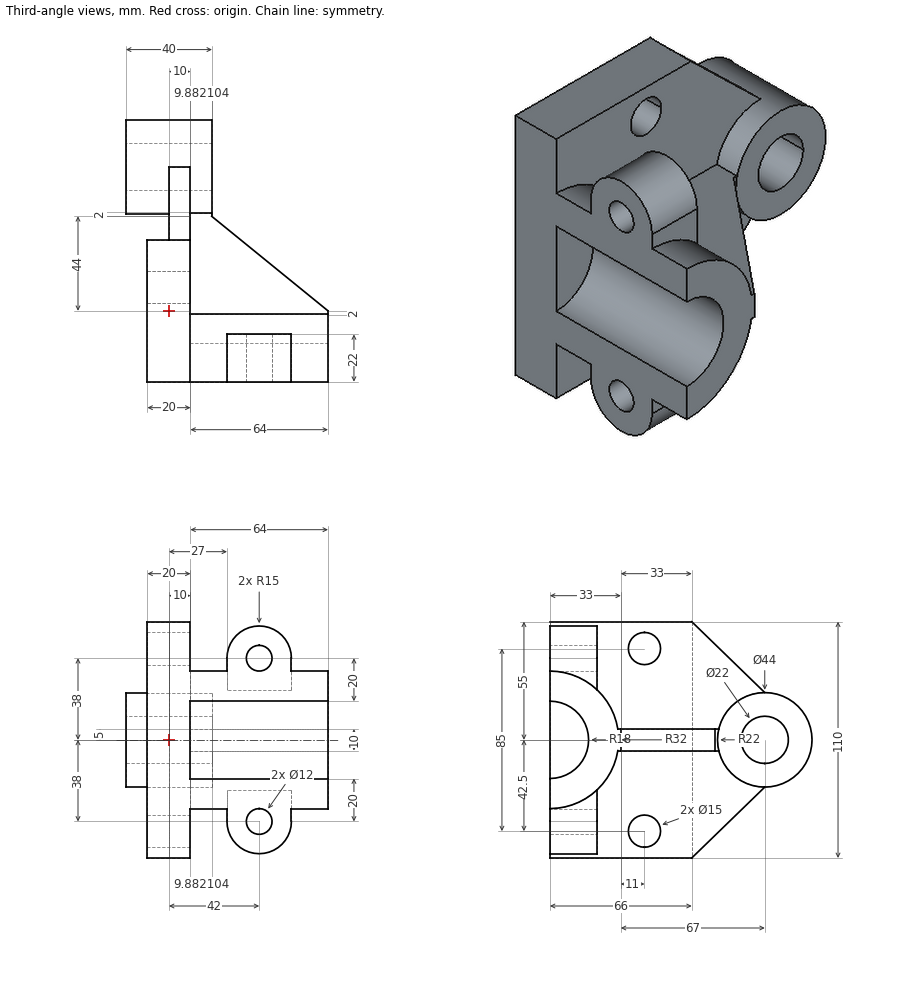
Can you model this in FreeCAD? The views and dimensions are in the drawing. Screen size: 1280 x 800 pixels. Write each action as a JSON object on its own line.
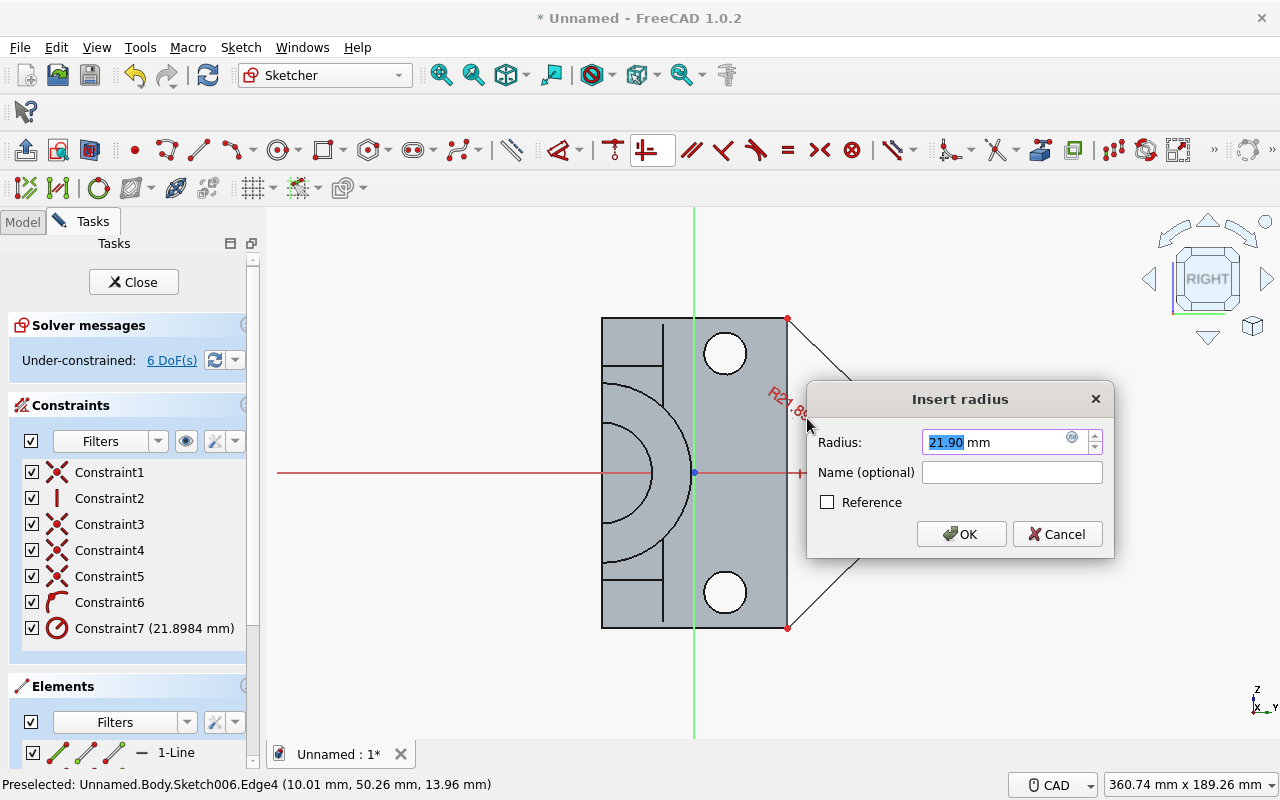
{"action": "type", "text": "22"}
{"action": "key", "text": "Return"}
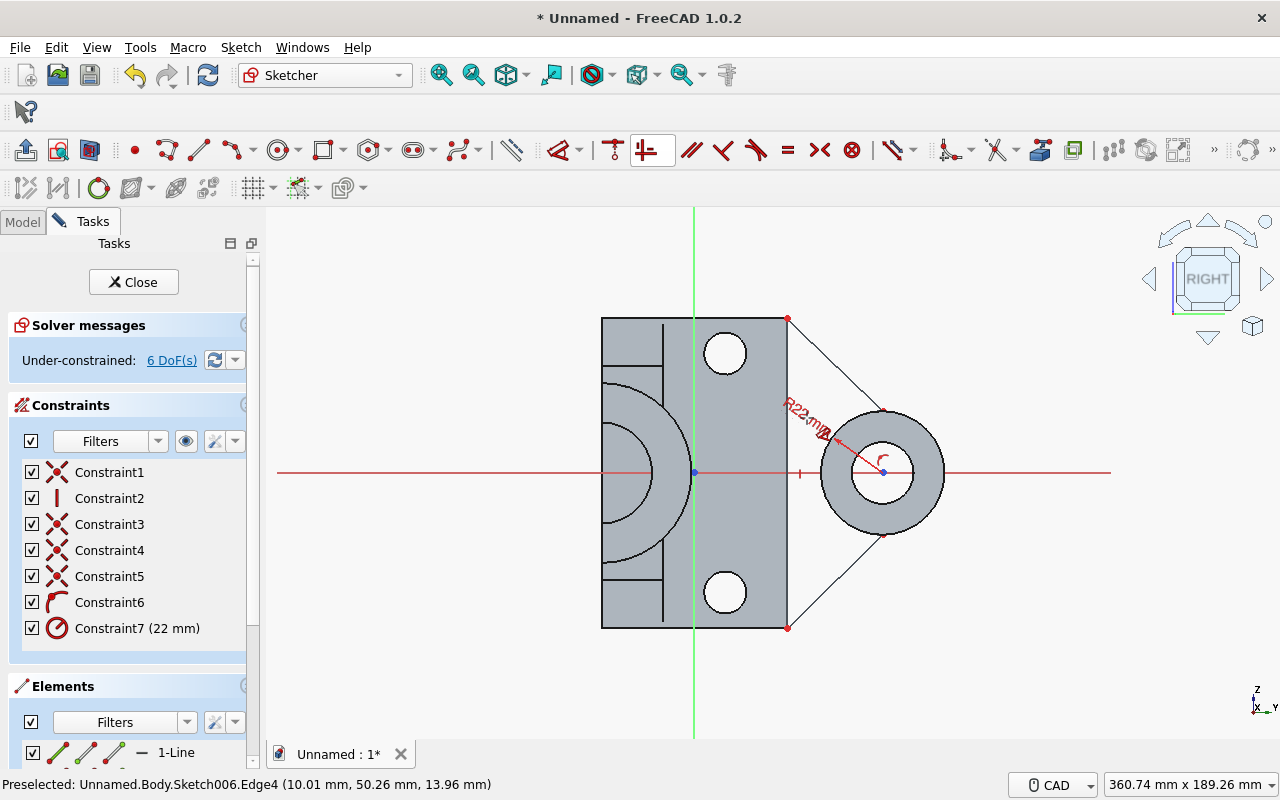
{"action": "left_click", "coordinate": [787, 412]}
{"action": "left_click", "coordinate": [753, 545]}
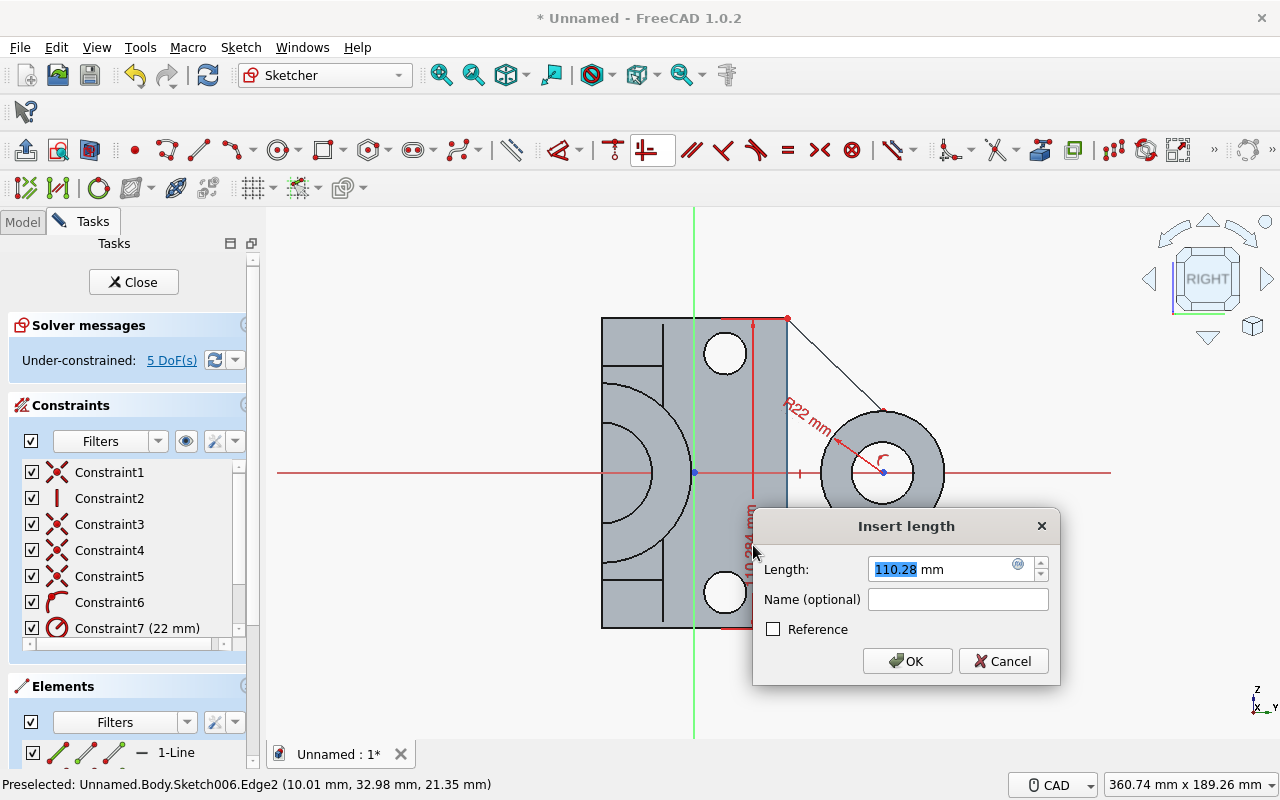
{"action": "type", "text": "110"}
{"action": "key", "text": "Return"}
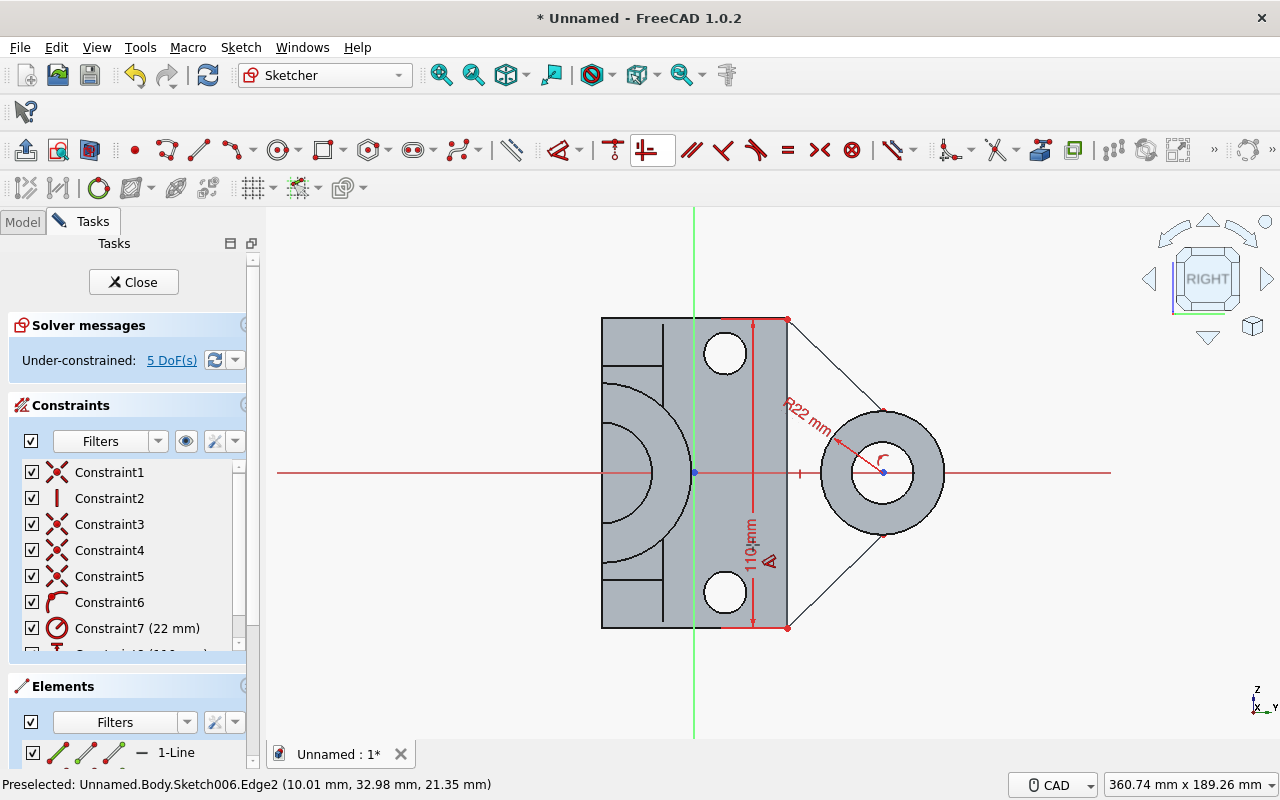
{"action": "left_click", "coordinate": [883, 411]}
{"action": "left_click", "coordinate": [745, 377]}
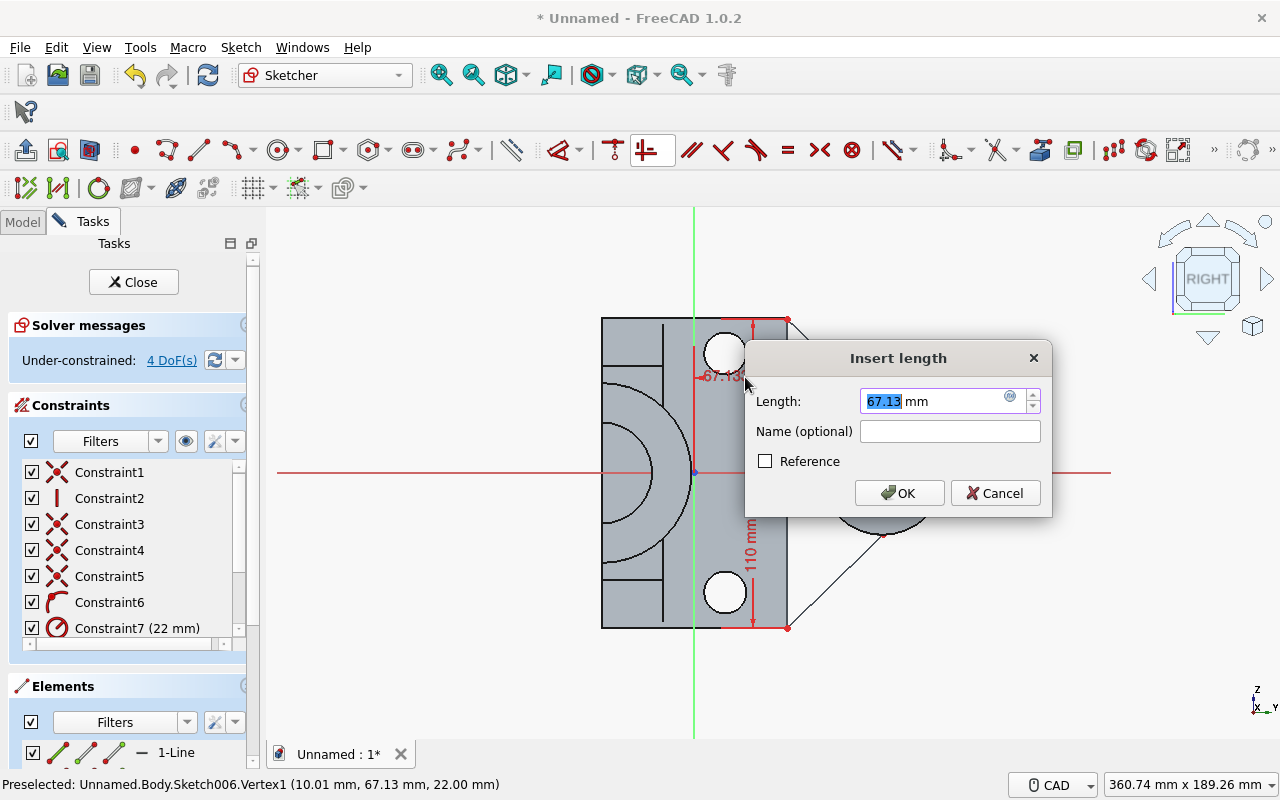
{"action": "type", "text": "67"}
{"action": "key", "text": "Return"}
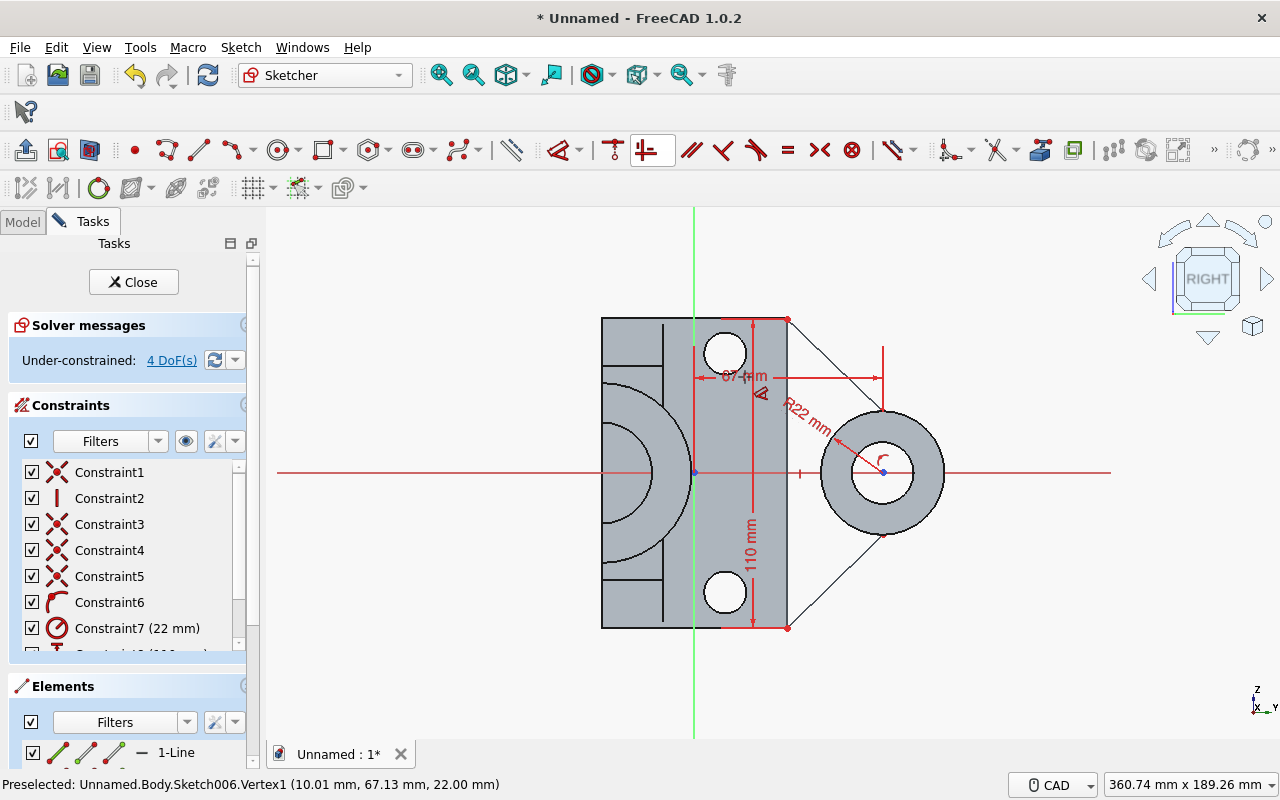
{"action": "left_click", "coordinate": [787, 319]}
{"action": "left_click", "coordinate": [741, 285]}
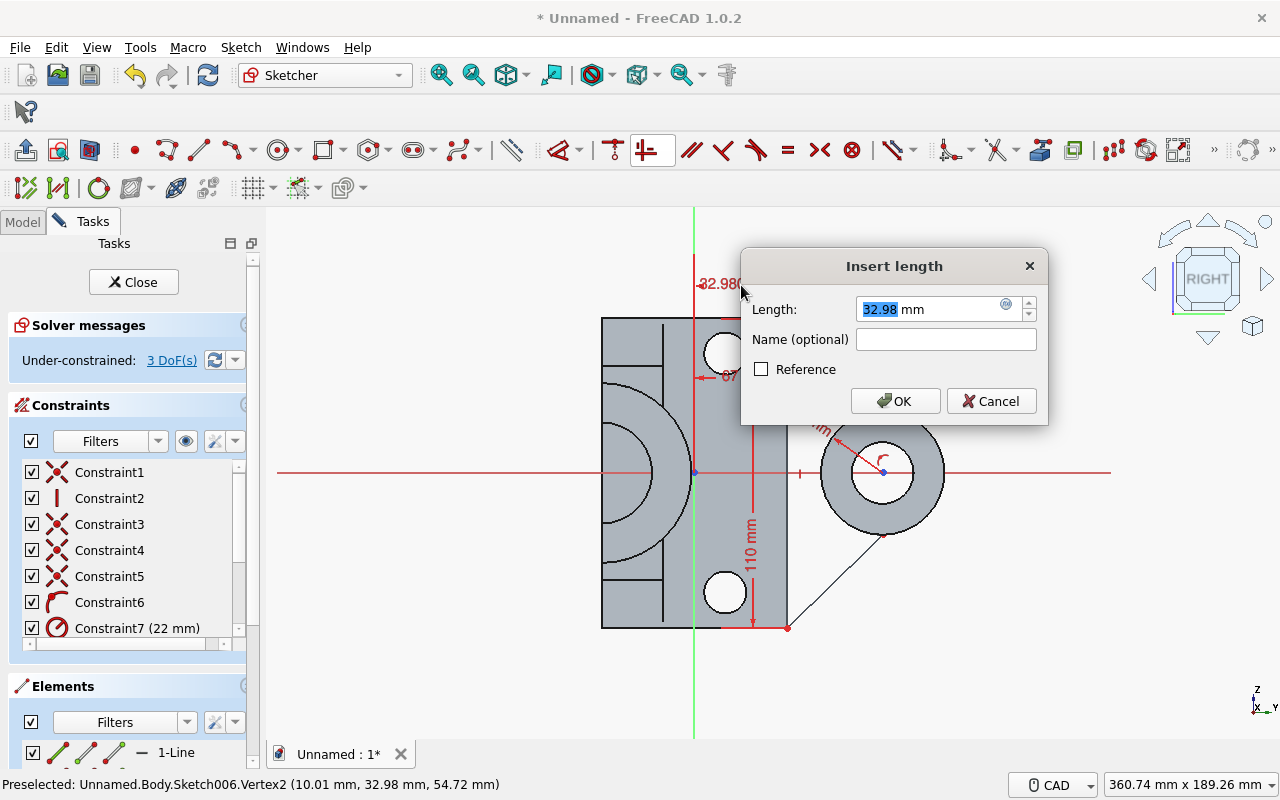
{"action": "type", "text": "33"}
{"action": "key", "text": "Return"}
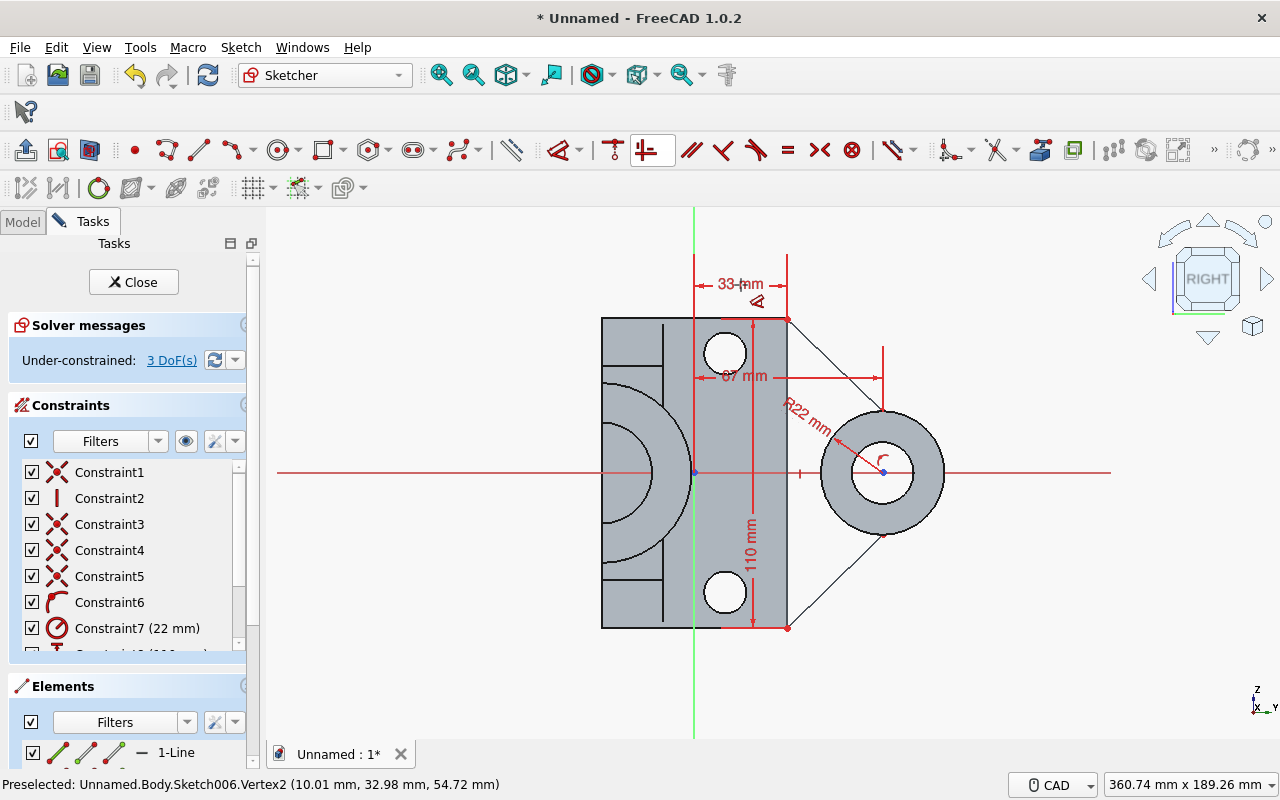
{"action": "left_click", "coordinate": [787, 319]}
{"action": "left_click", "coordinate": [660, 396]}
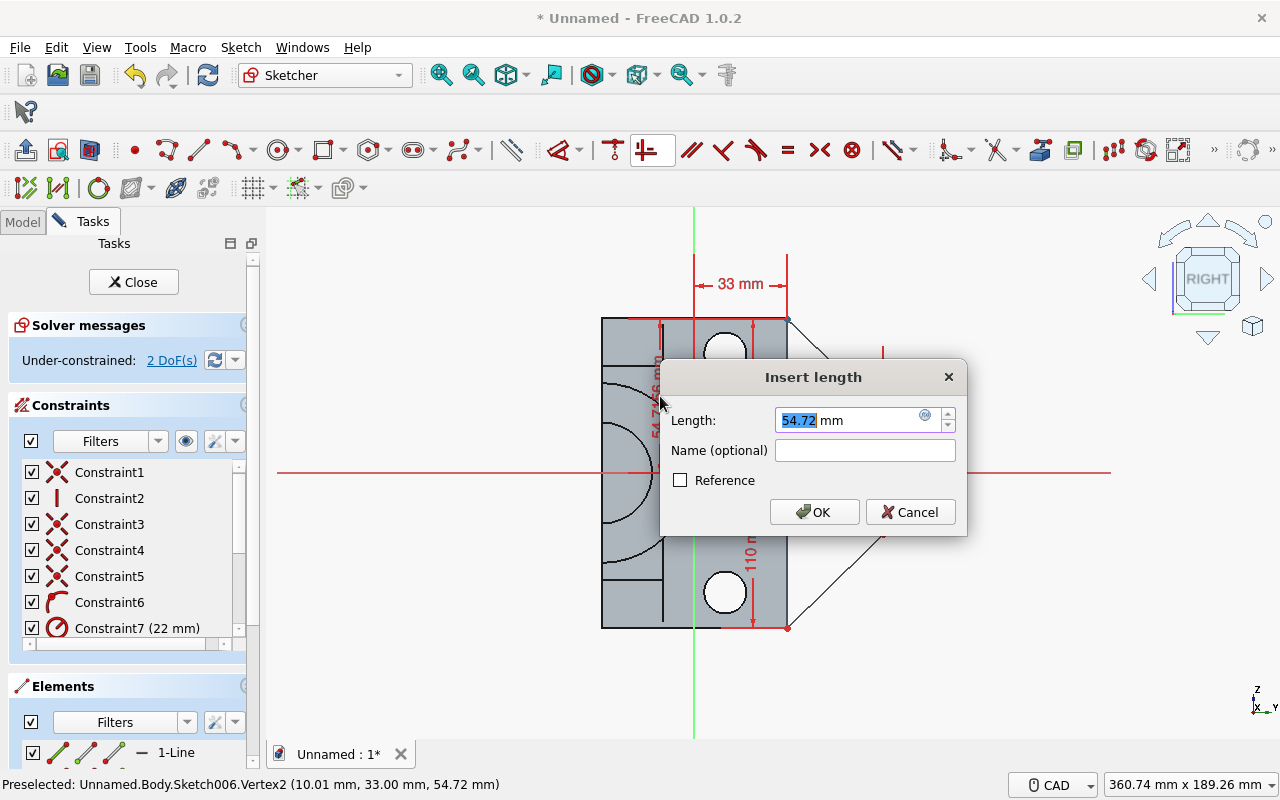
{"action": "type", "text": "55"}
{"action": "key", "text": "Return"}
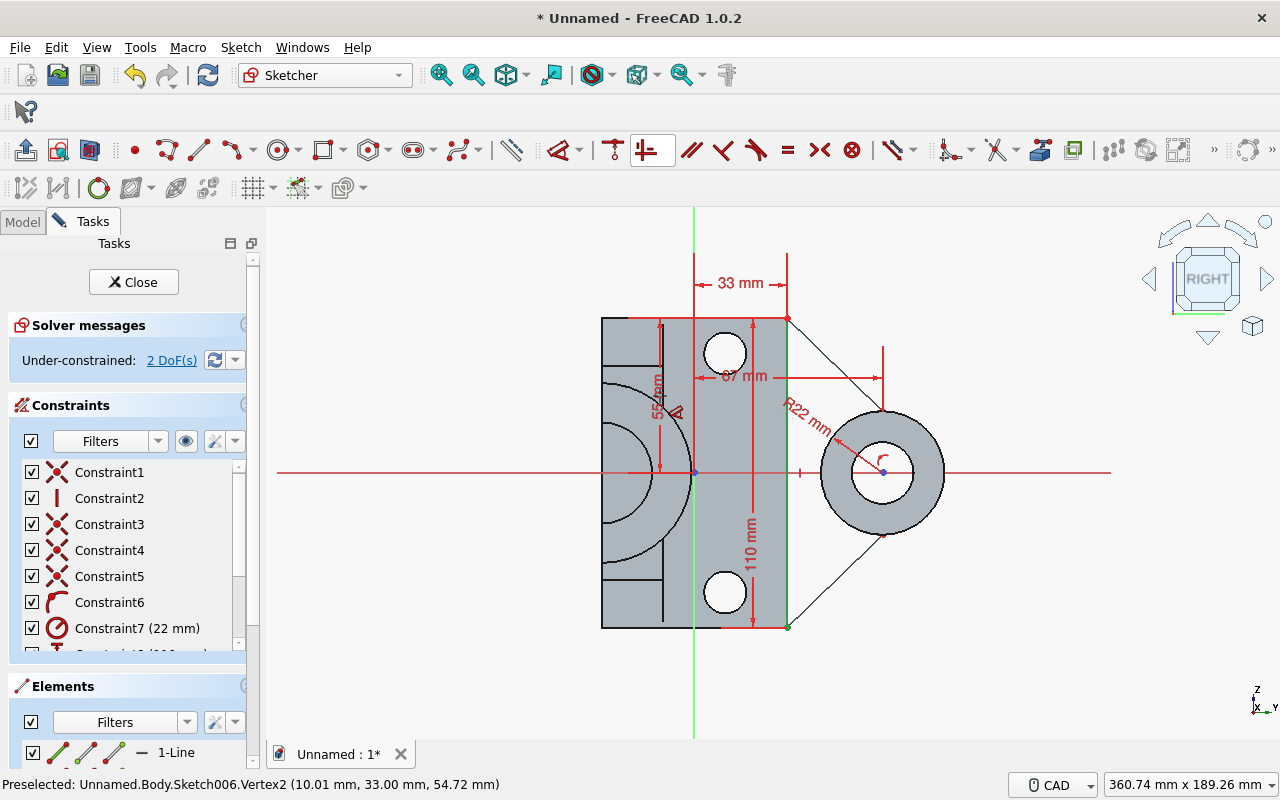
{"action": "left_click", "coordinate": [883, 535]}
{"action": "left_click", "coordinate": [745, 569]}